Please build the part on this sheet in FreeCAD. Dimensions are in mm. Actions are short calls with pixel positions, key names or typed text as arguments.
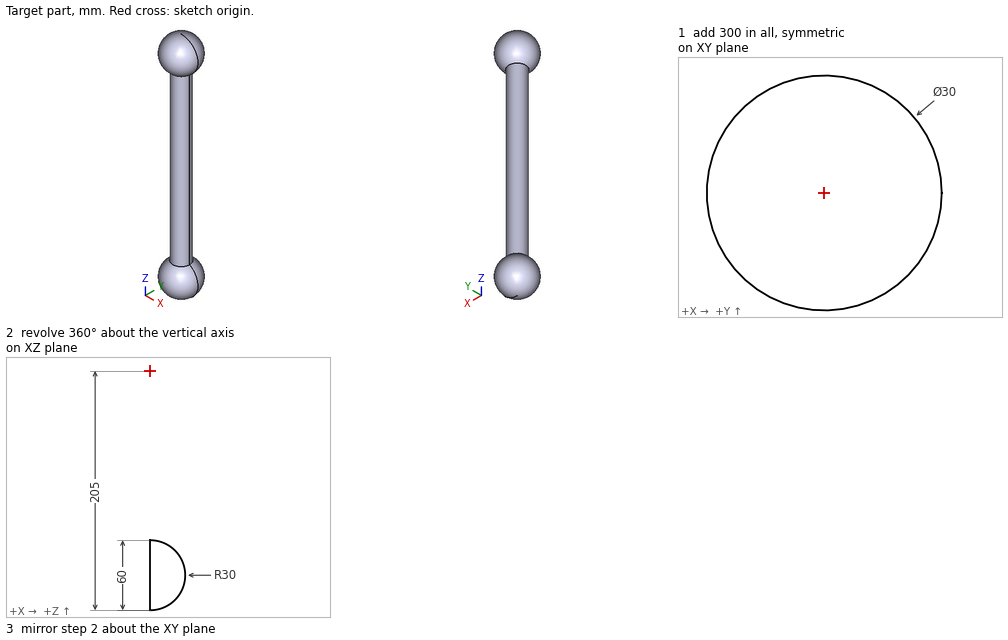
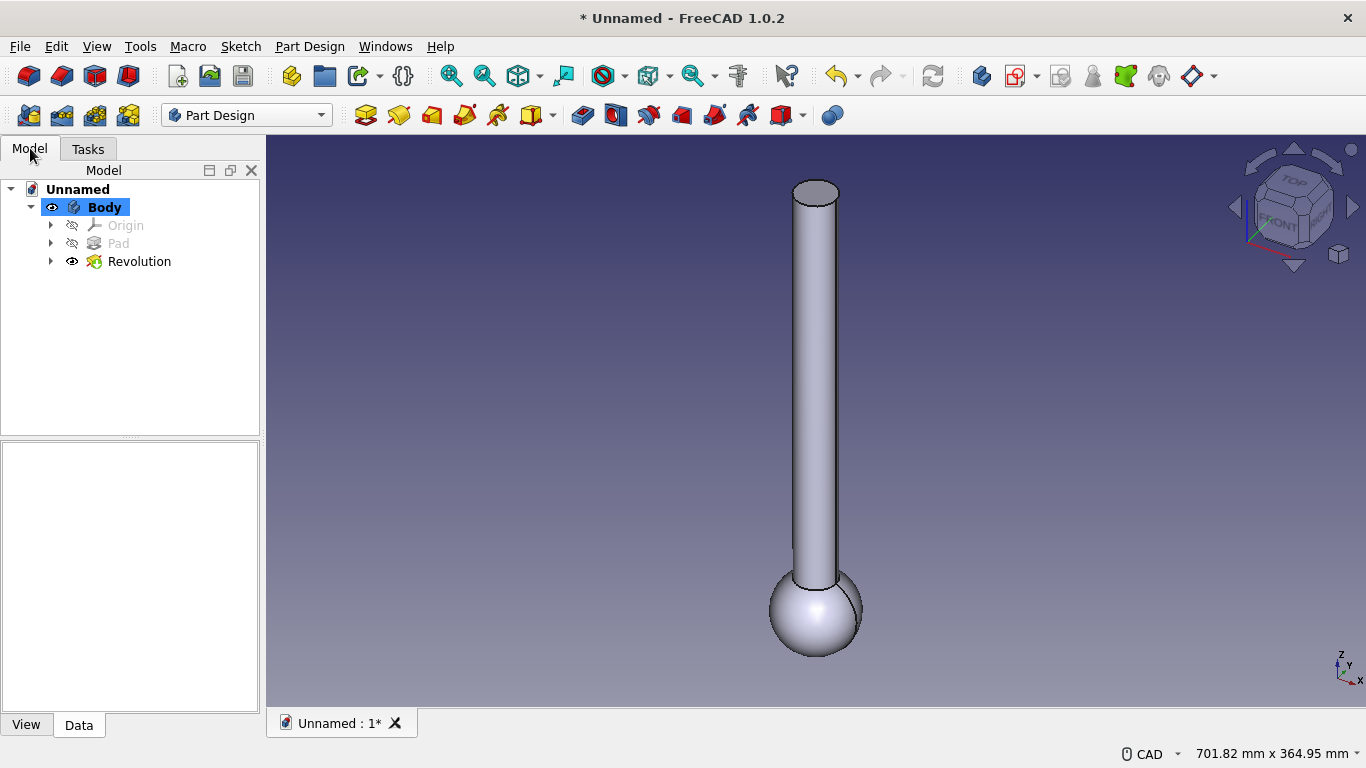
click(117, 261)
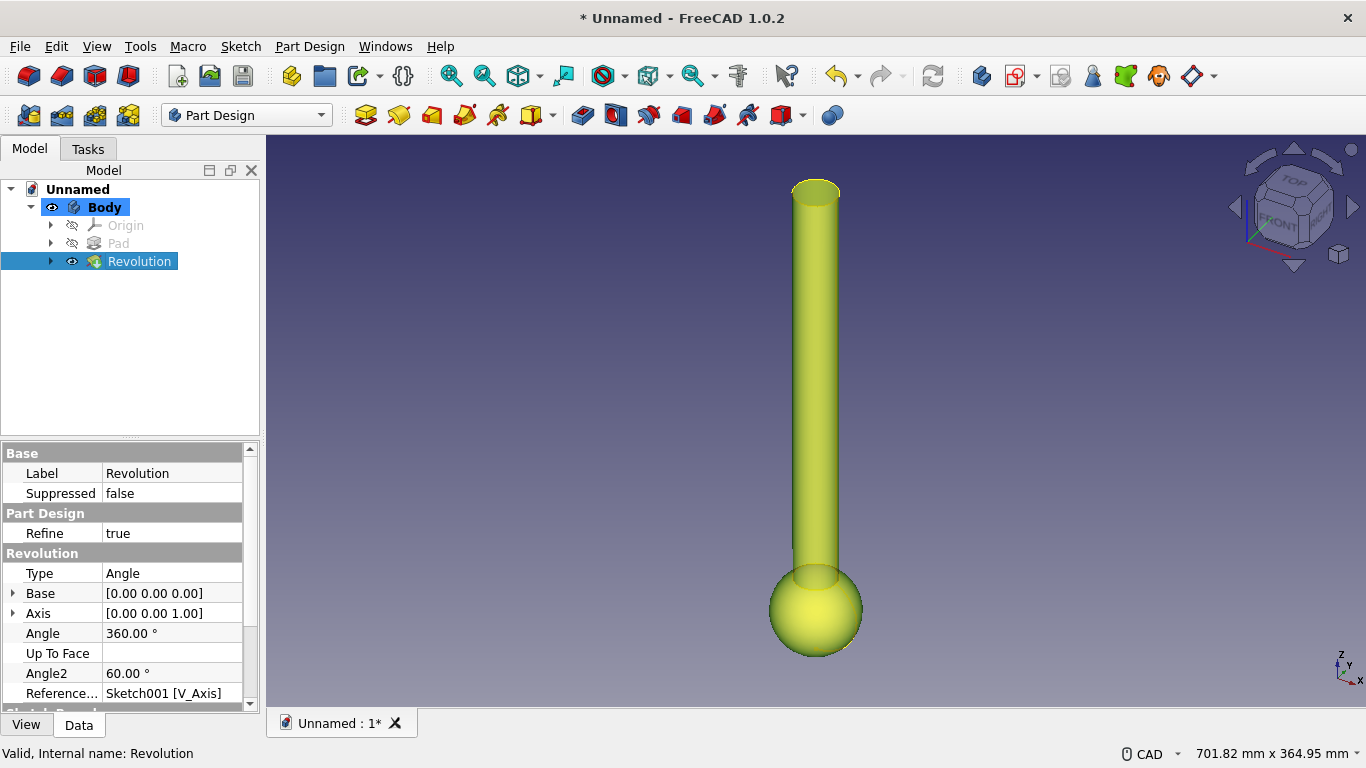
click(29, 116)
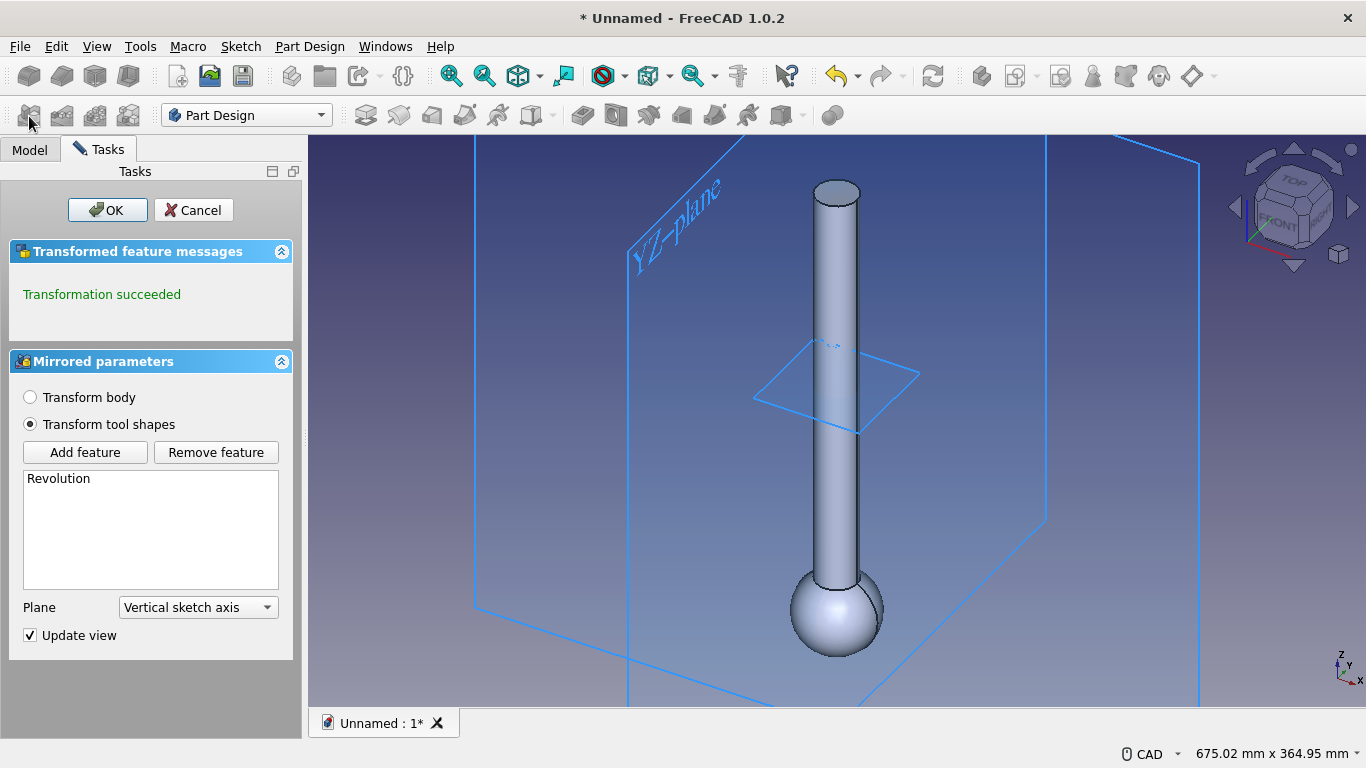
click(199, 608)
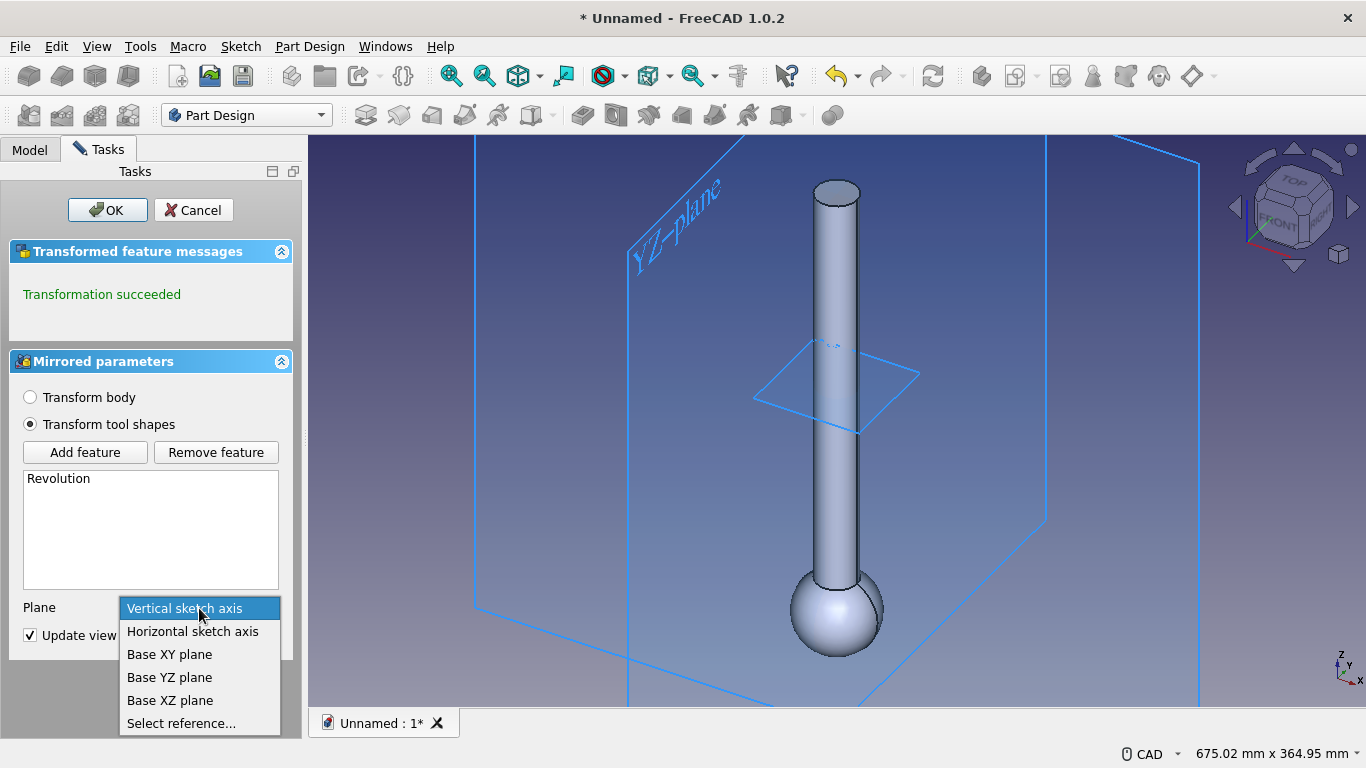
click(198, 654)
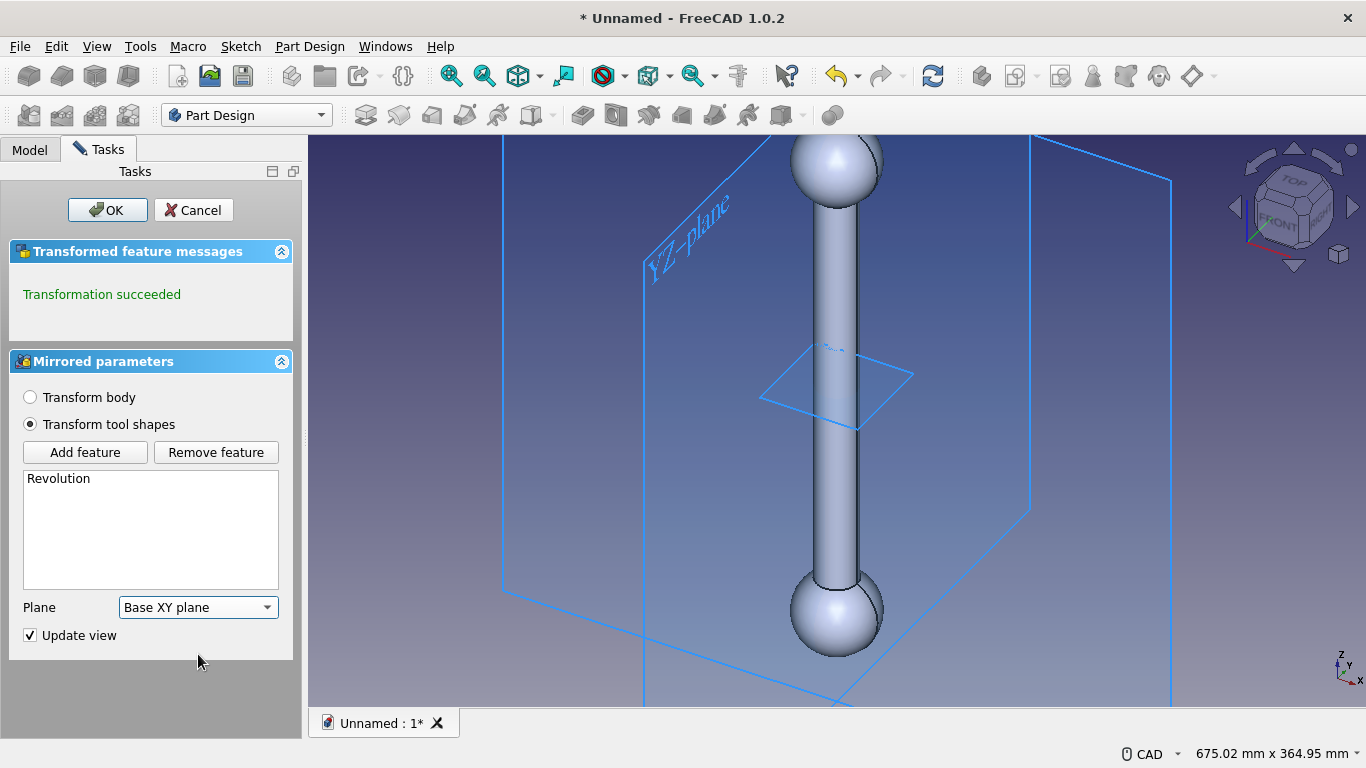
click(108, 210)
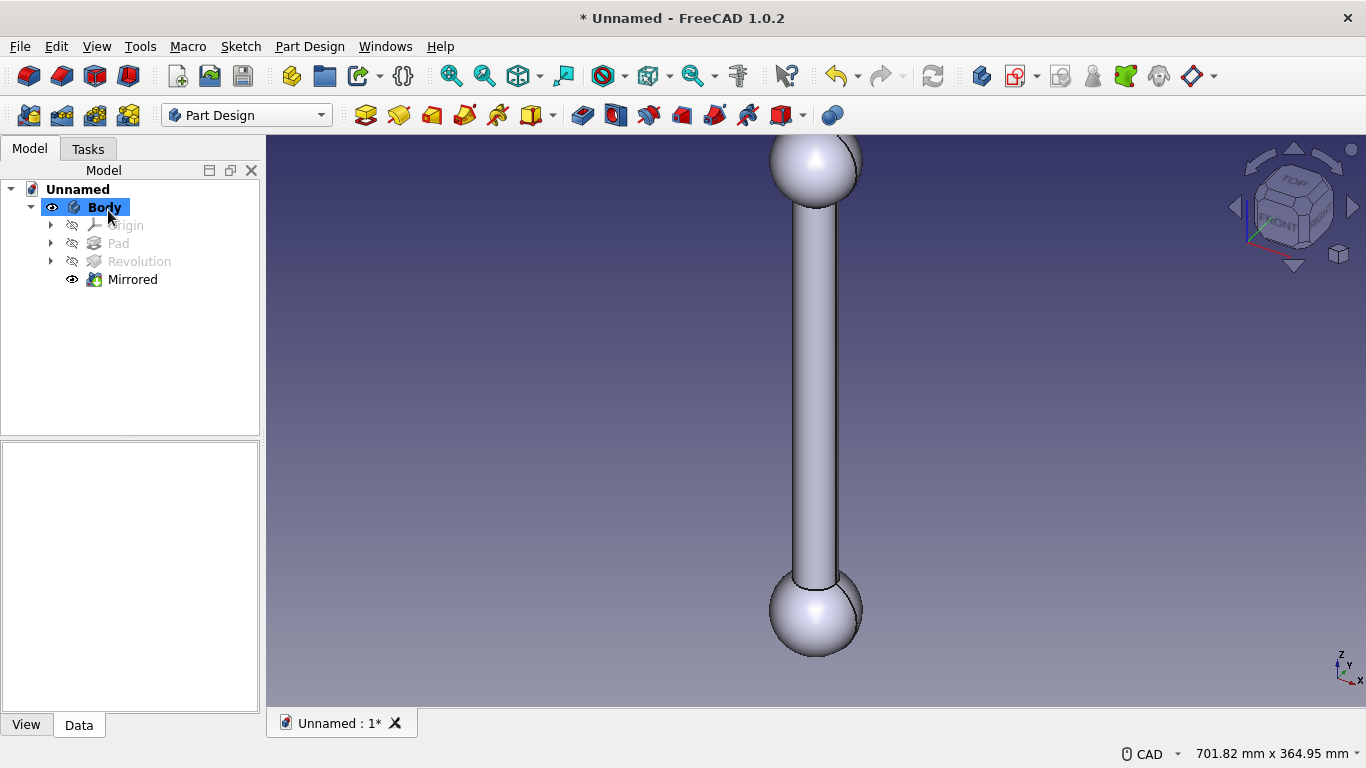
key(0)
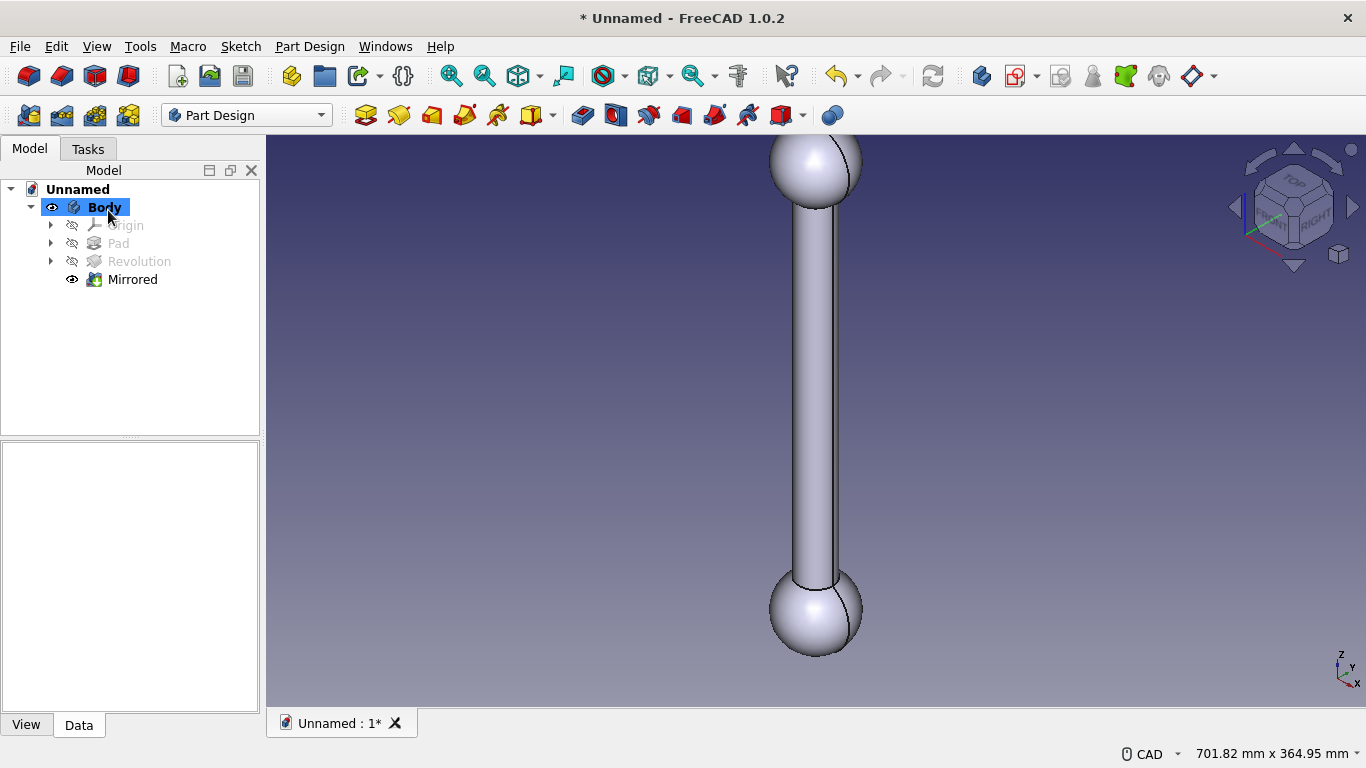
click(452, 76)